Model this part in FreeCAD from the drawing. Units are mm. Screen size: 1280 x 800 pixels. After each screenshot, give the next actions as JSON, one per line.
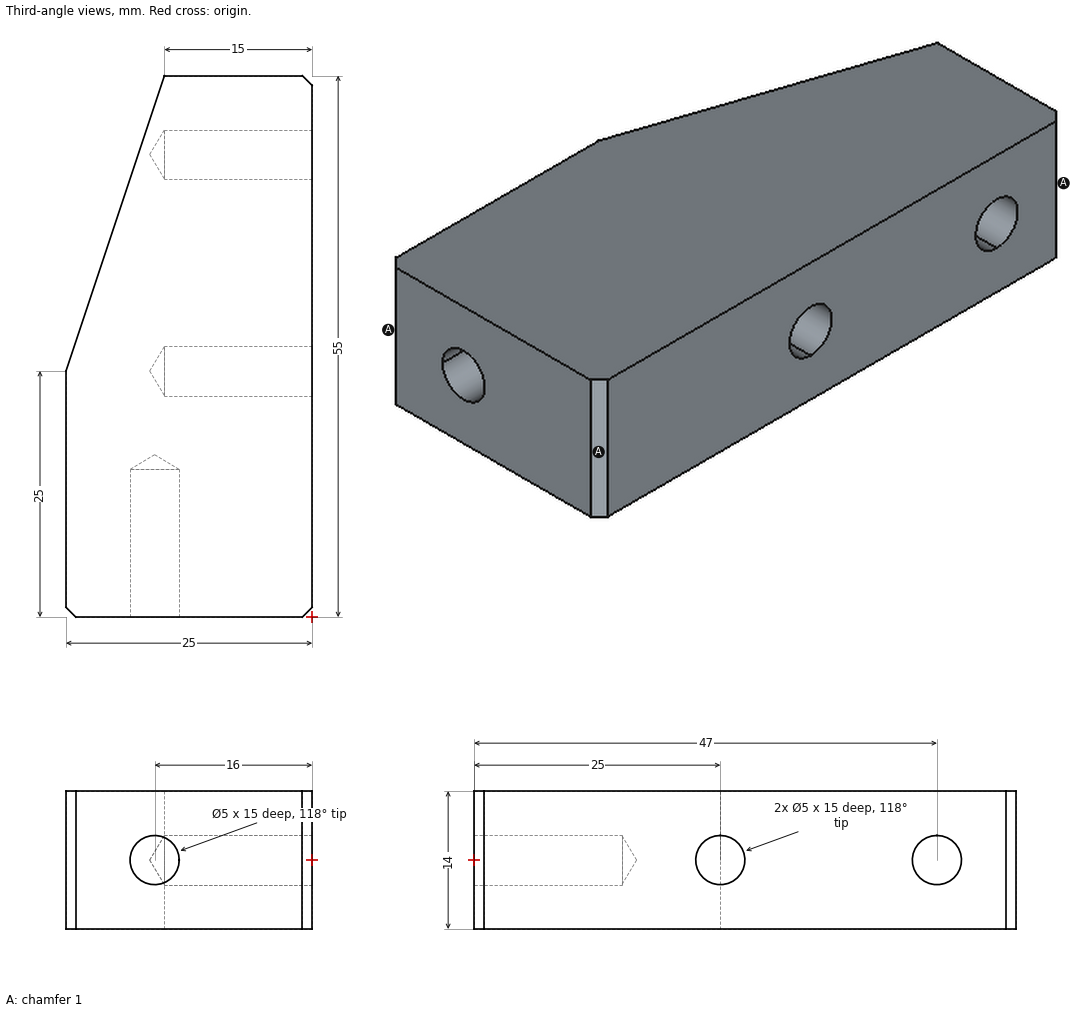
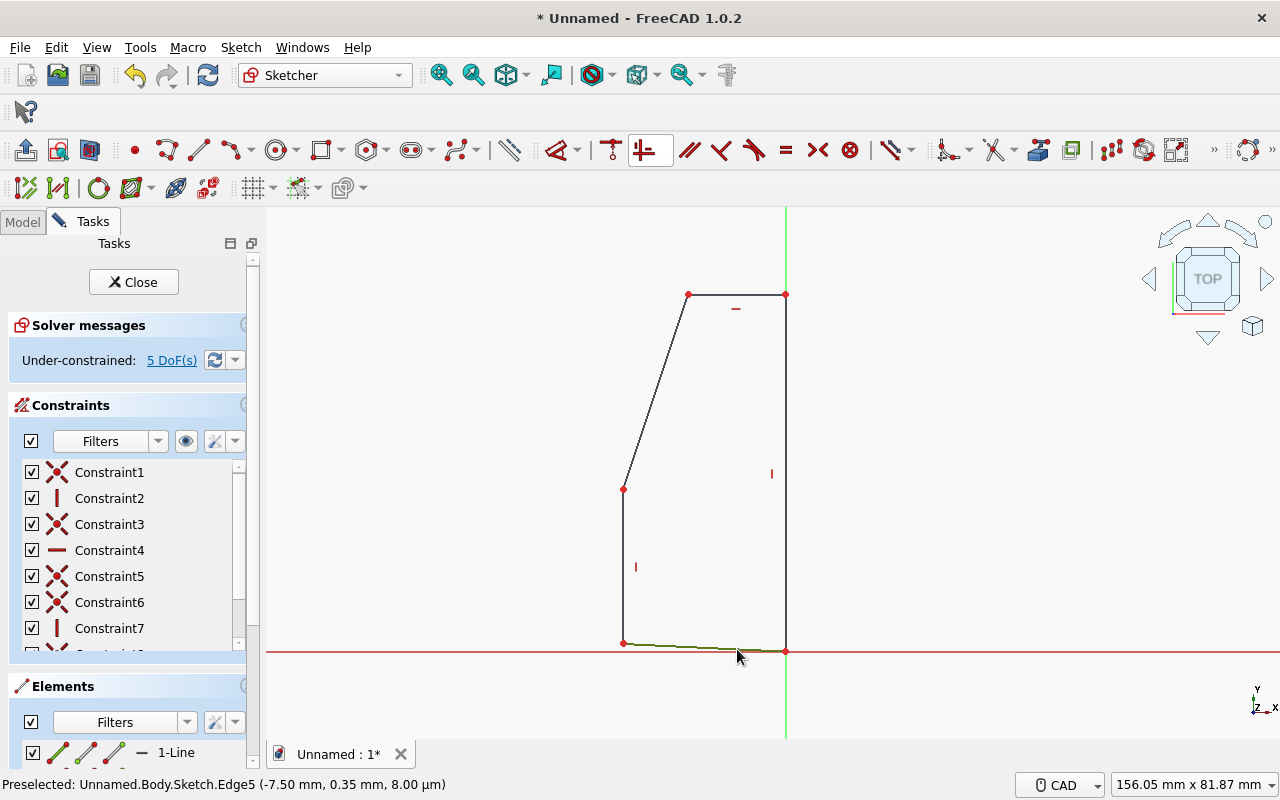
{"action": "key", "text": "h"}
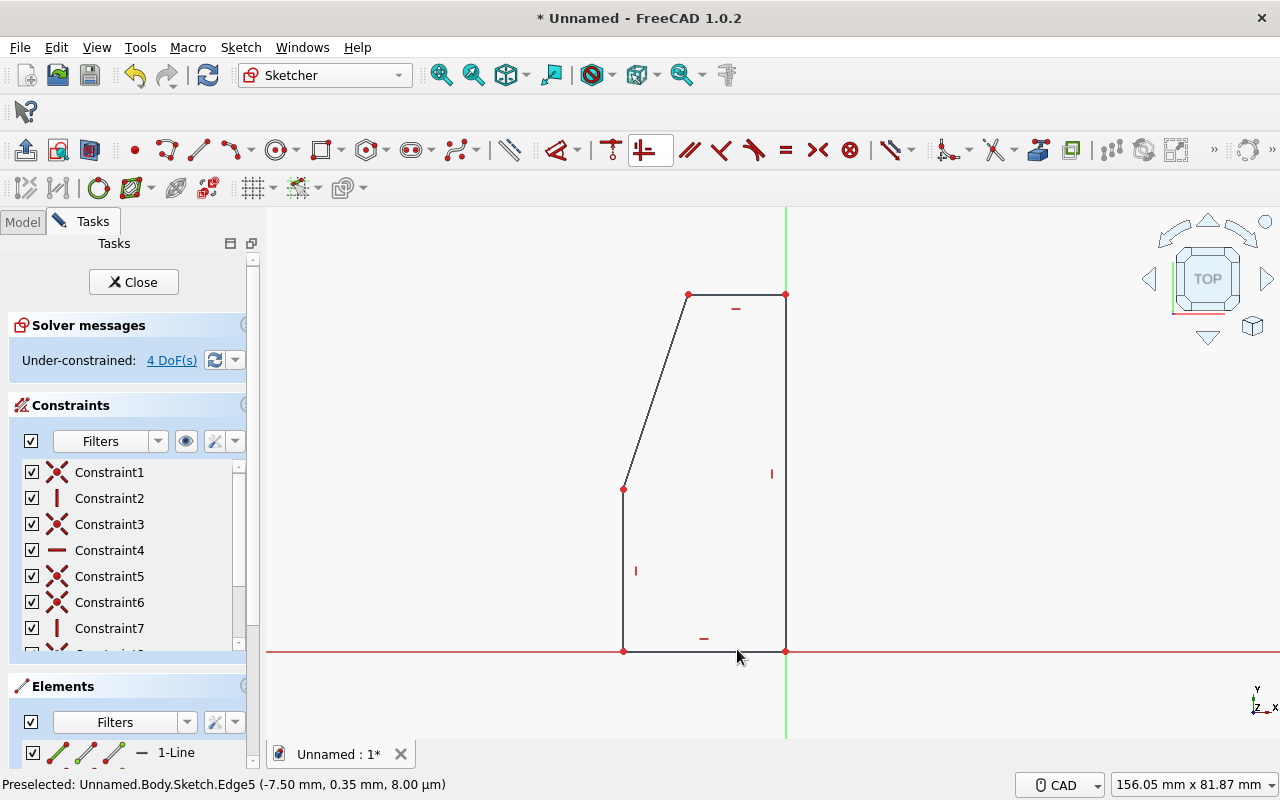
{"action": "key", "text": "d"}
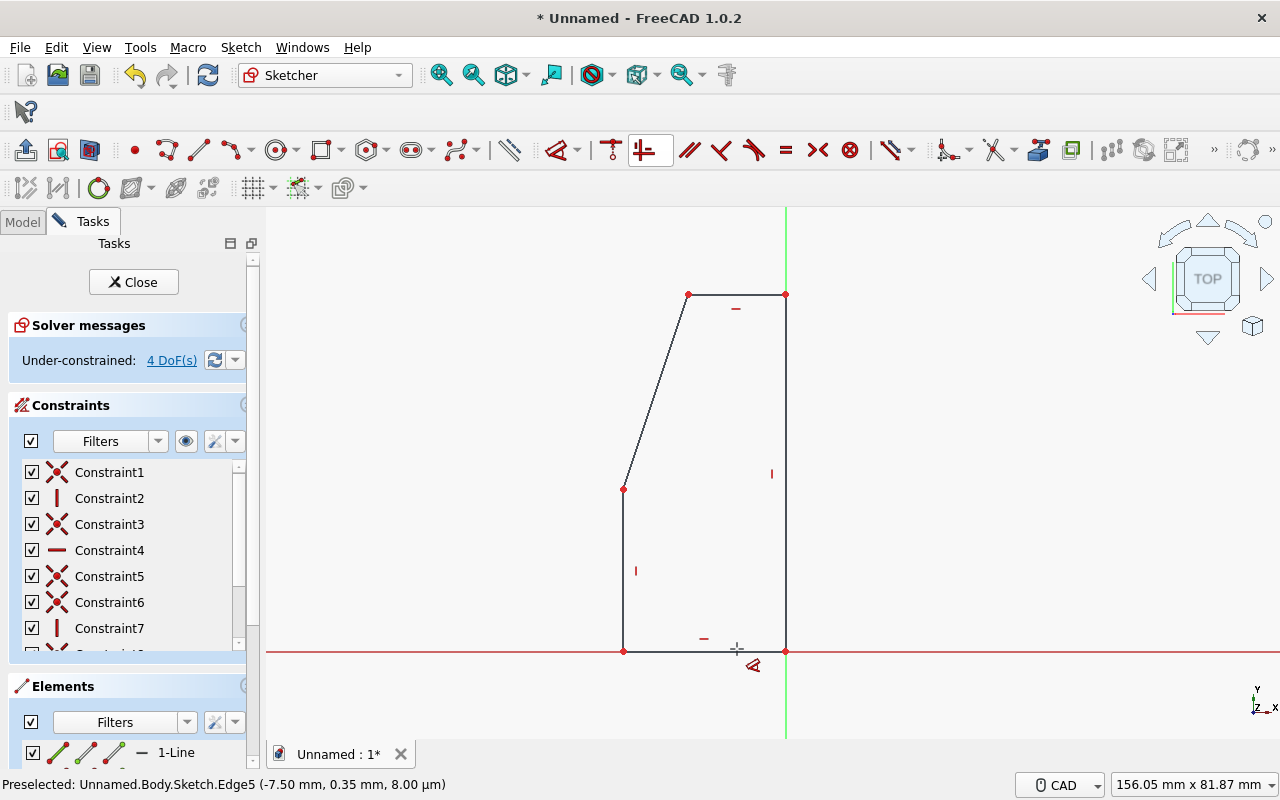
{"action": "left_click", "coordinate": [786, 545]}
{"action": "left_click", "coordinate": [820, 473]}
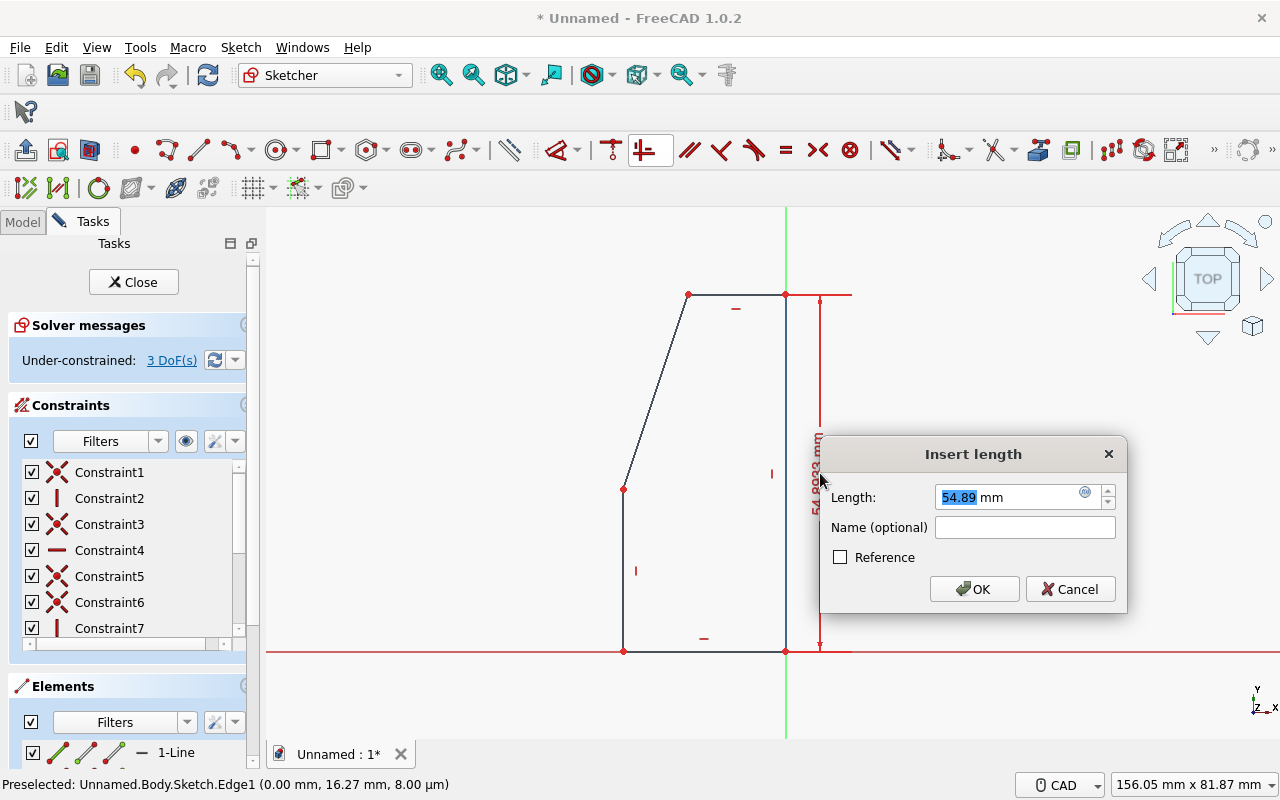
{"action": "type", "text": "55"}
{"action": "key", "text": "Return"}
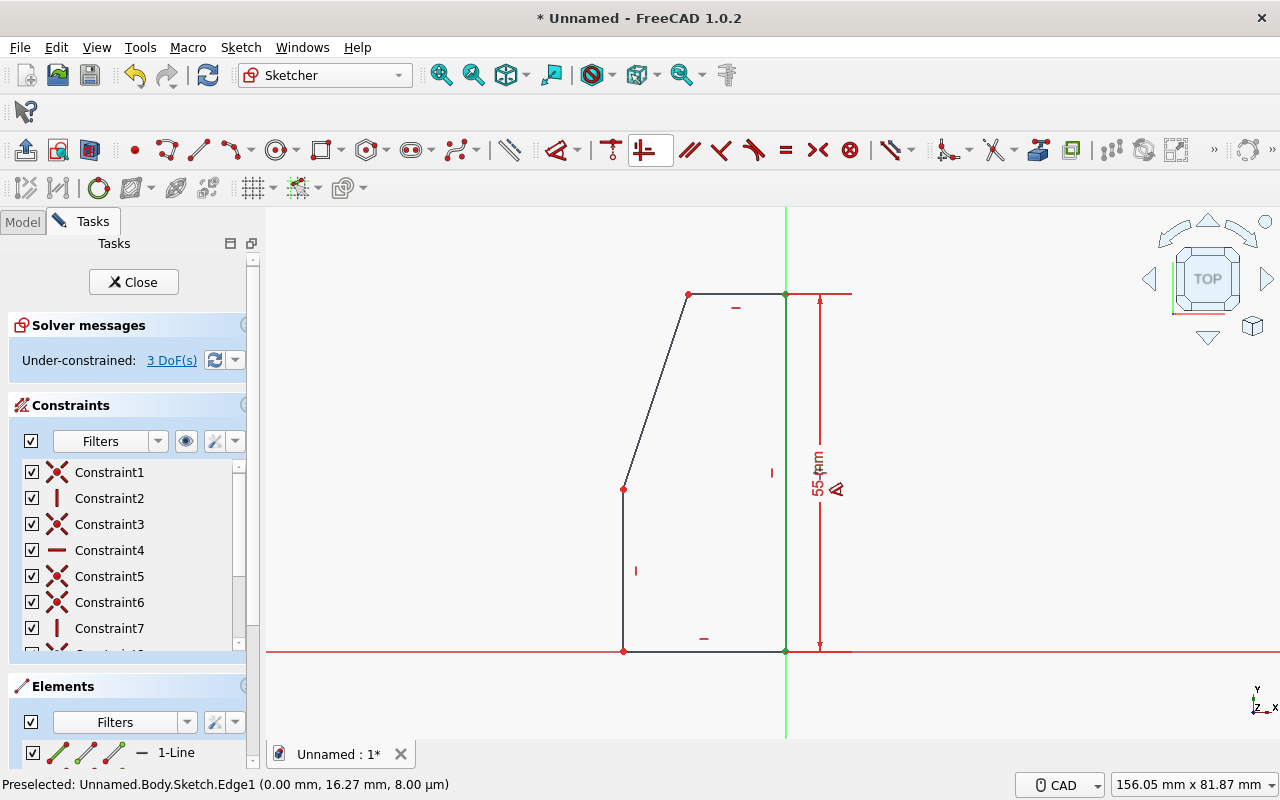
{"action": "left_click", "coordinate": [756, 294]}
{"action": "left_click", "coordinate": [737, 260]}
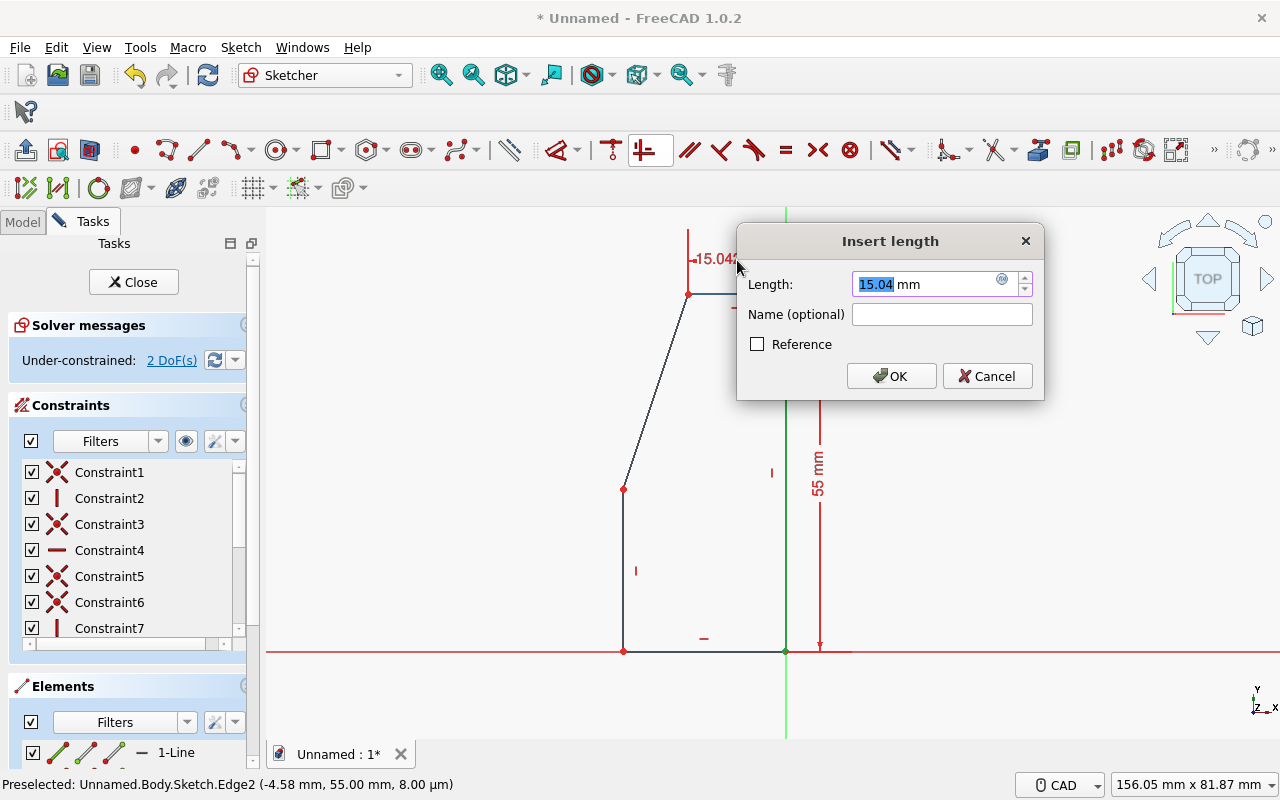
{"action": "type", "text": "15"}
{"action": "key", "text": "Return"}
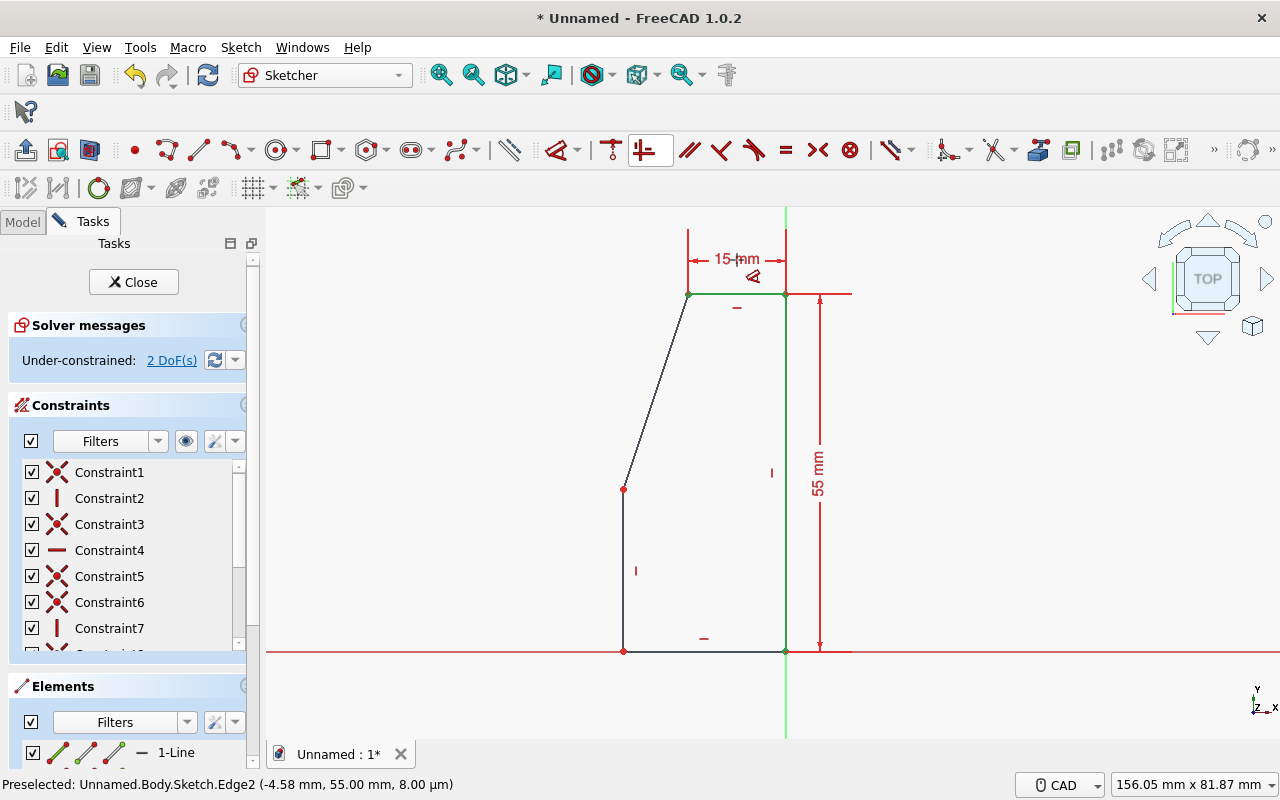
{"action": "left_click", "coordinate": [623, 539]}
{"action": "left_click", "coordinate": [589, 571]}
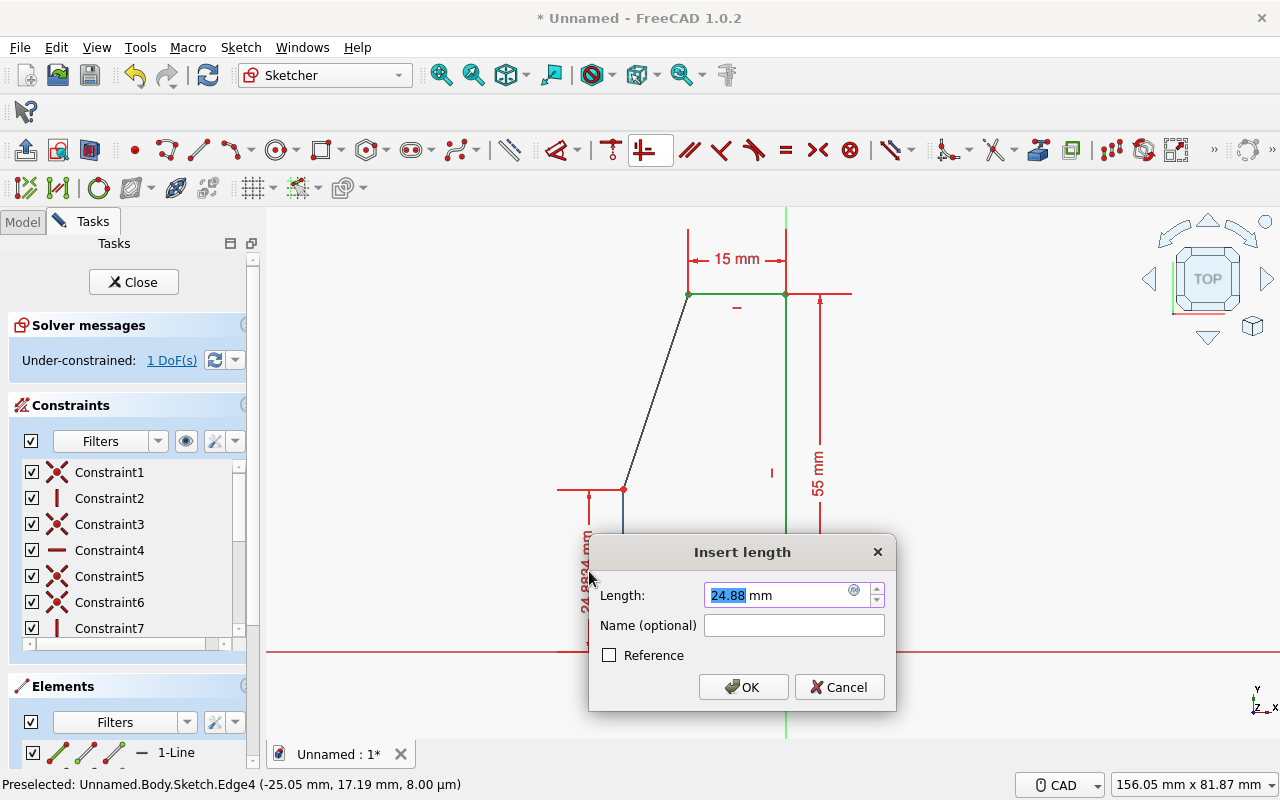
{"action": "type", "text": "25"}
{"action": "key", "text": "Return"}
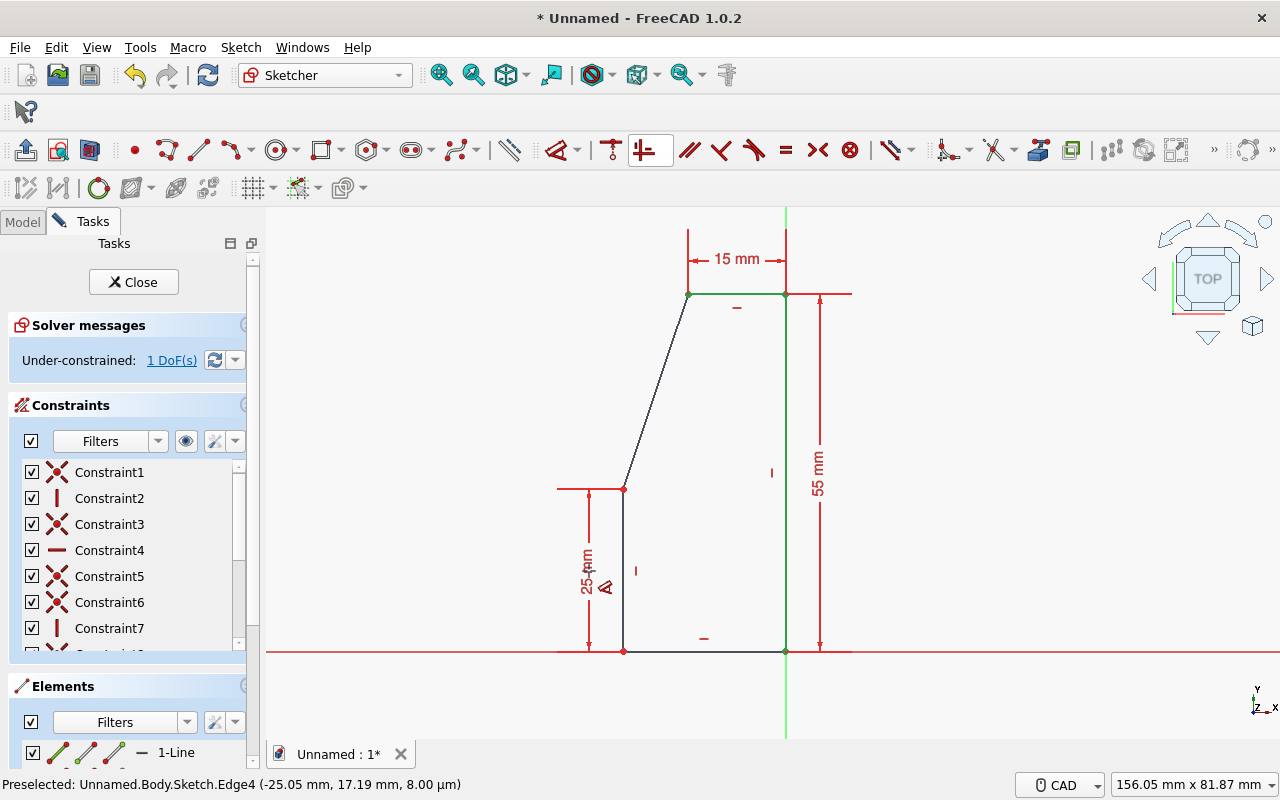
{"action": "left_click", "coordinate": [672, 652]}
{"action": "left_click", "coordinate": [704, 686]}